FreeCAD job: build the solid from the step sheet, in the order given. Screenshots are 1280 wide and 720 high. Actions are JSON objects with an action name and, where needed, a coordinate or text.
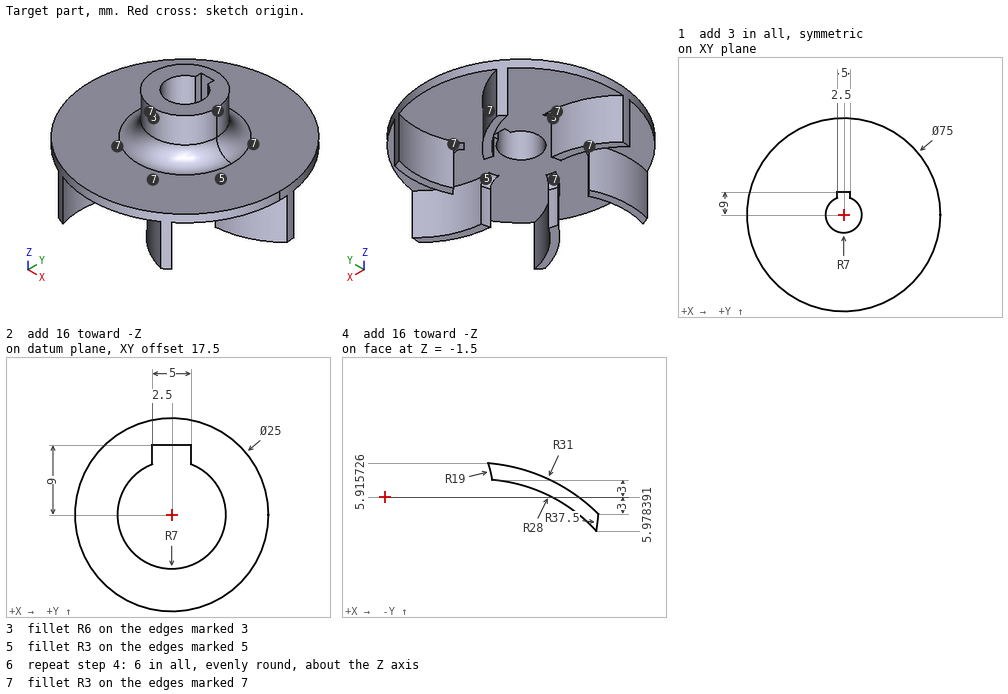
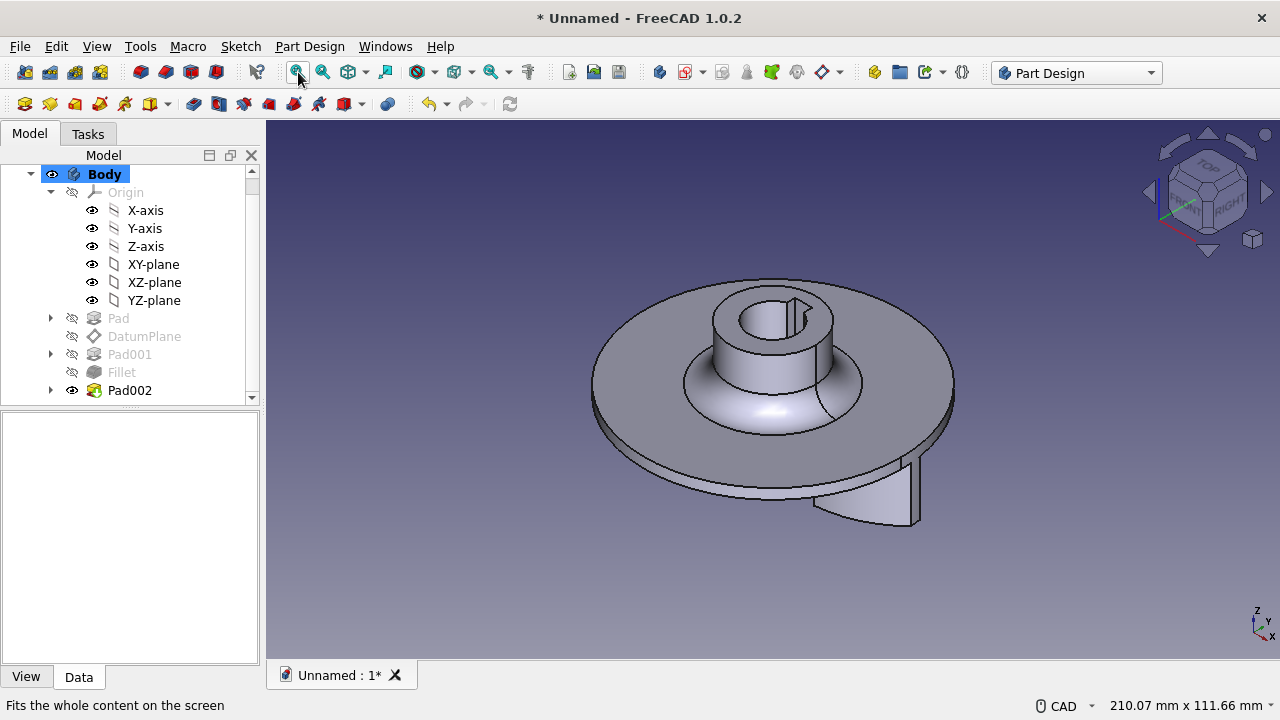
{"action": "key", "text": "2"}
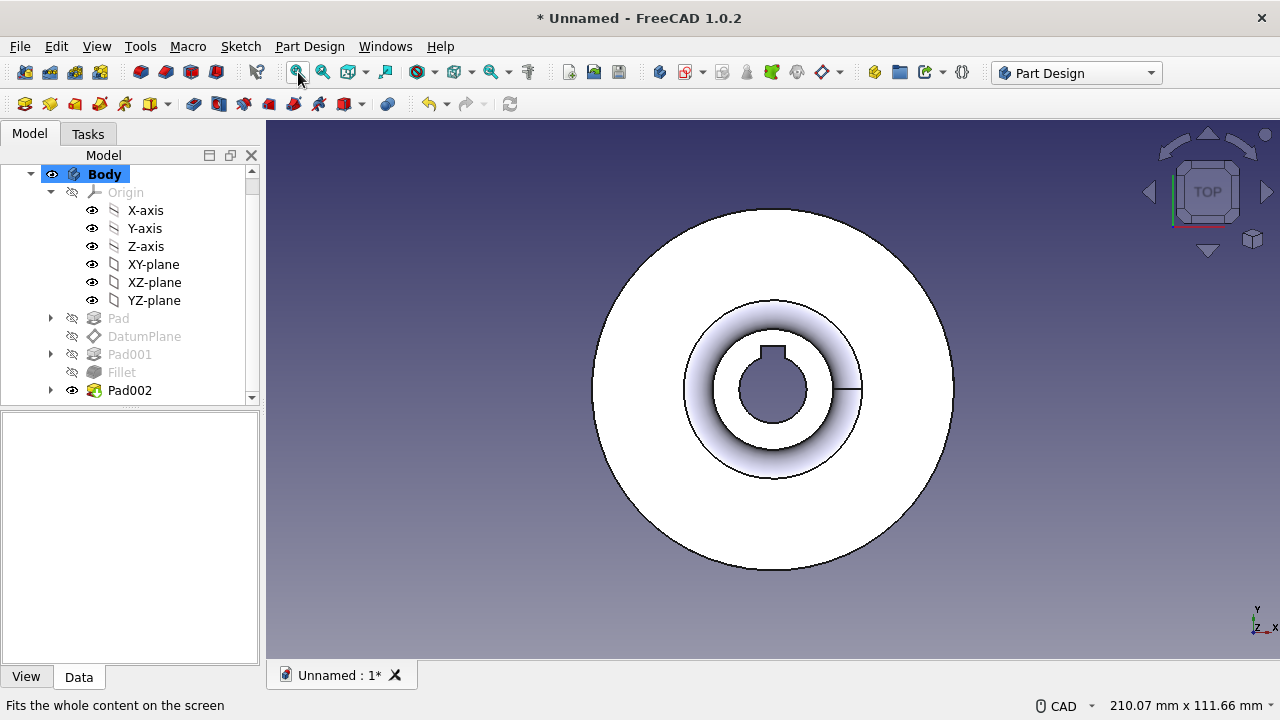
{"action": "scroll", "coordinate": [862, 410], "scroll_direction": "up", "scroll_amount": 6}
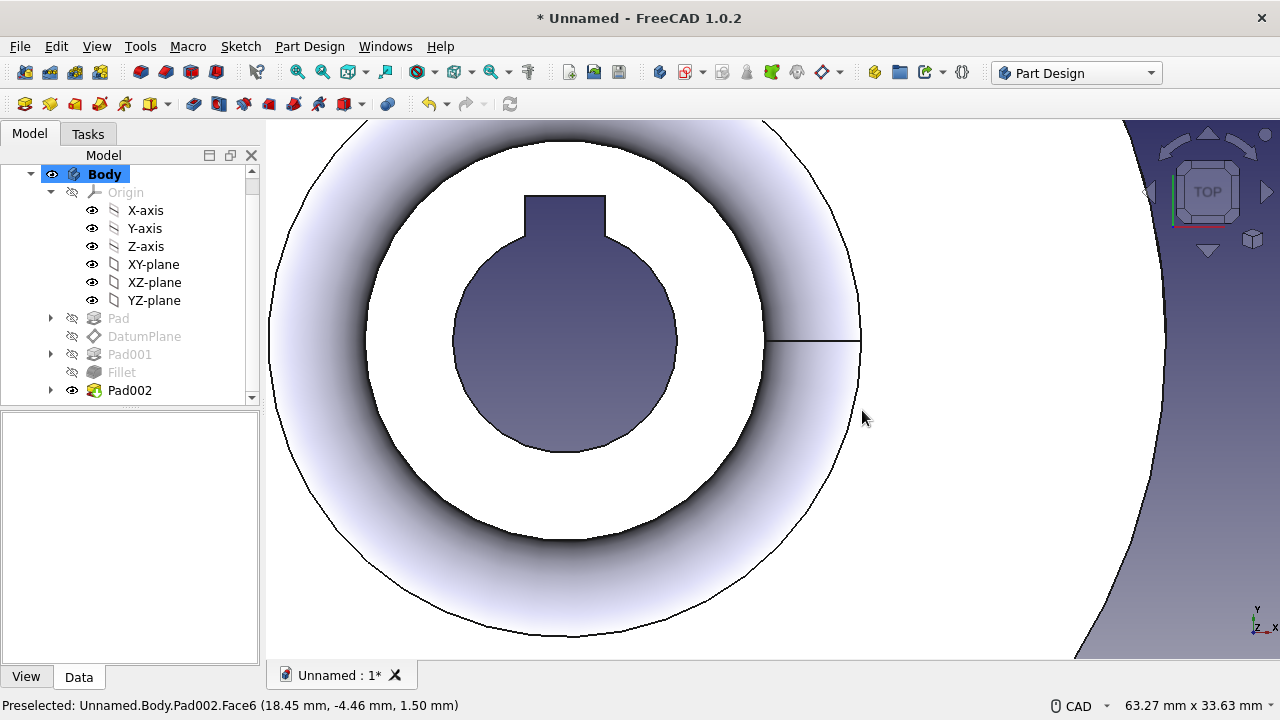
{"action": "left_click", "coordinate": [298, 72]}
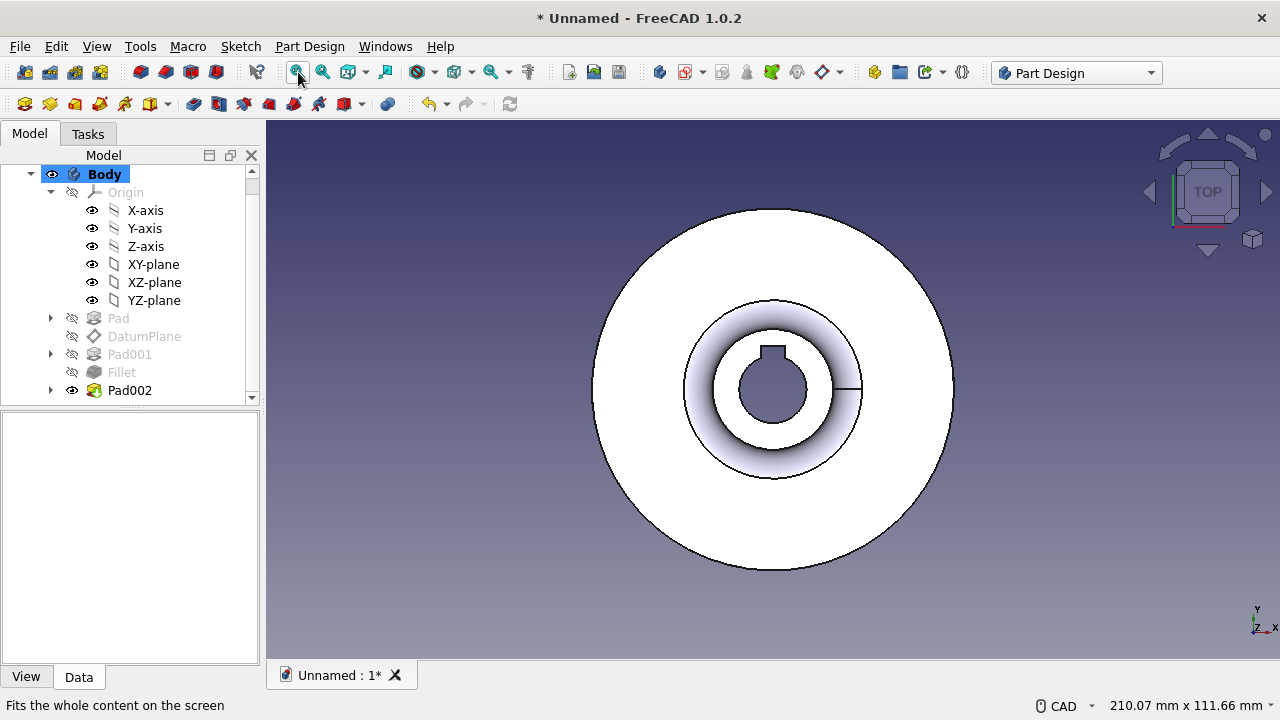
{"action": "key", "text": "1"}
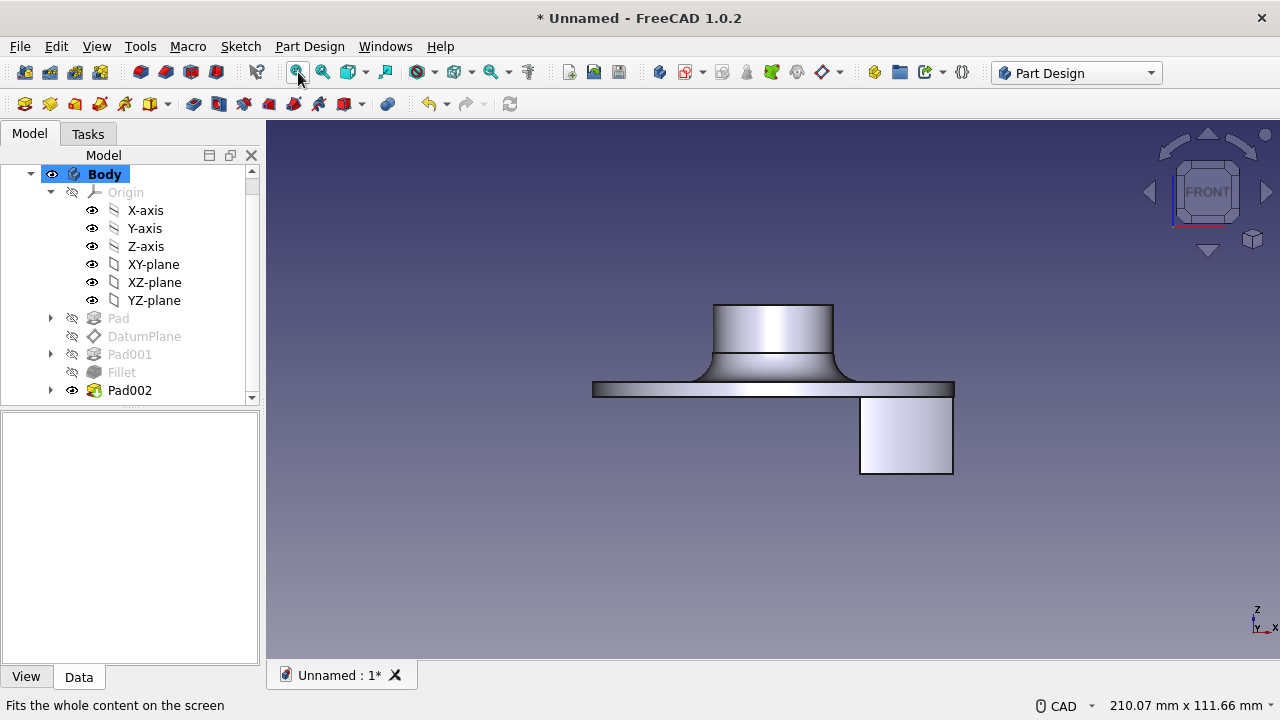
{"action": "left_click", "coordinate": [298, 72]}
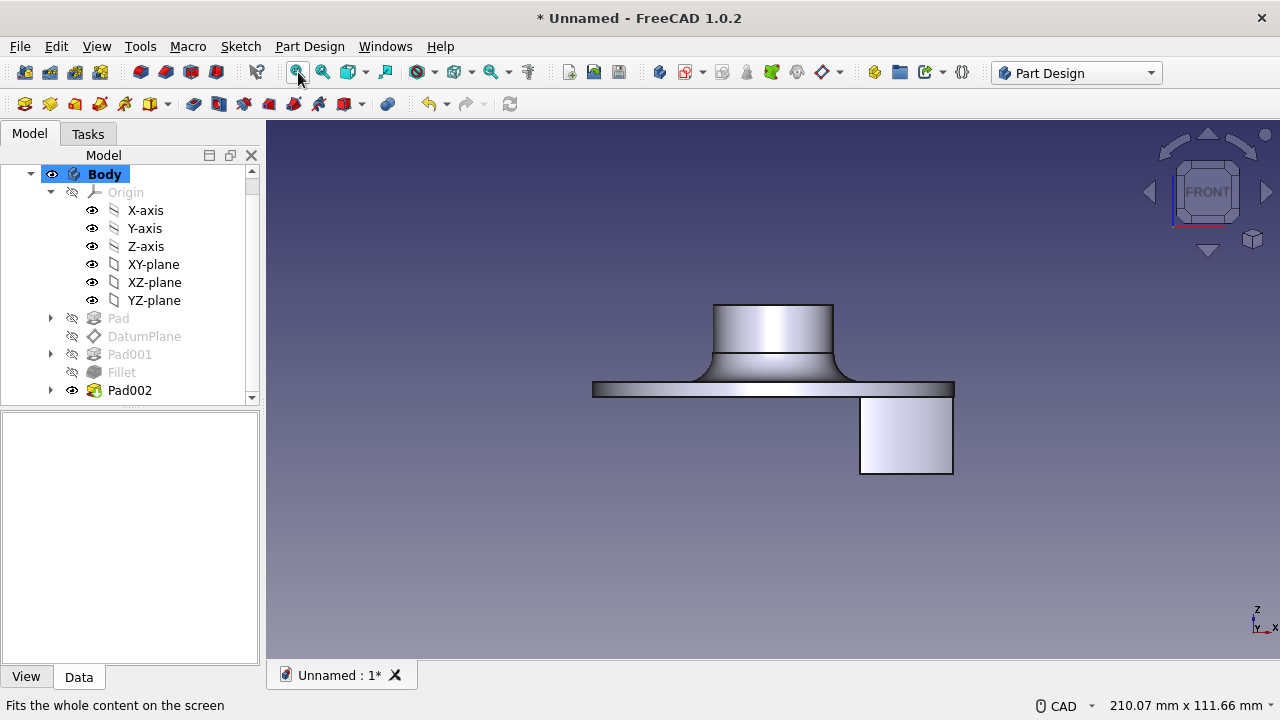
{"action": "scroll", "coordinate": [862, 396], "scroll_direction": "up", "scroll_amount": 6}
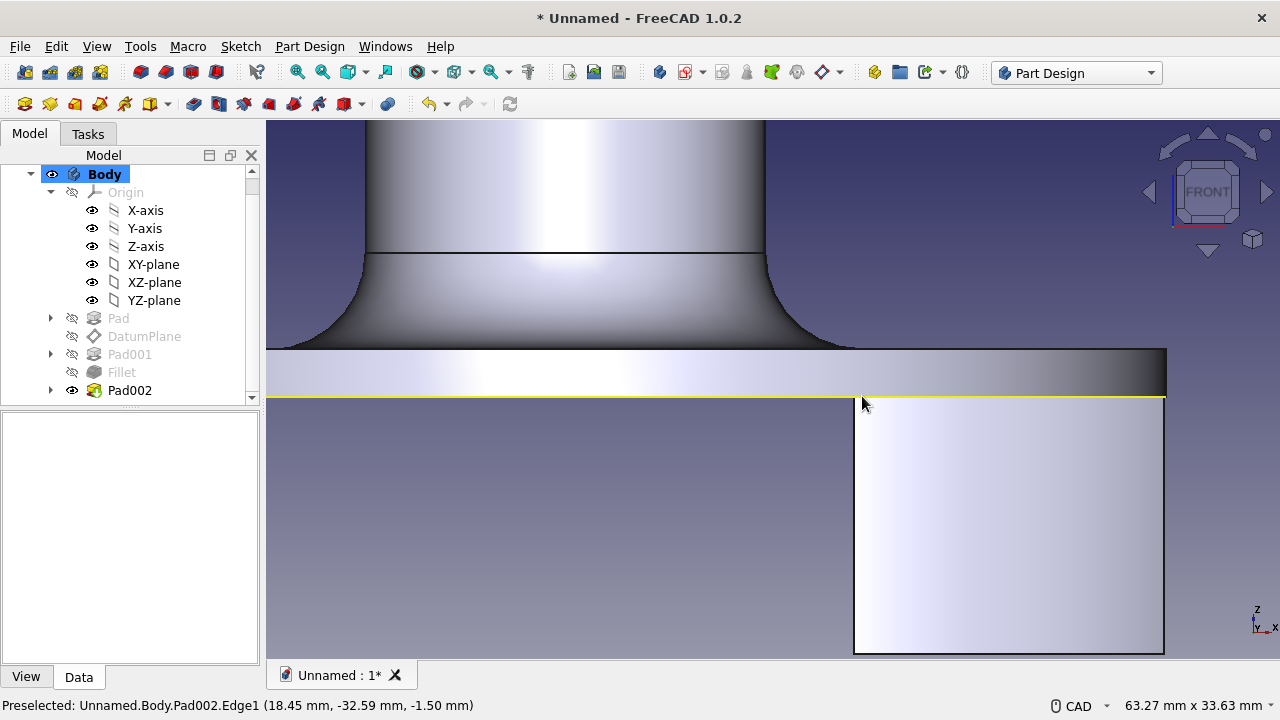
{"action": "key", "text": "v f"}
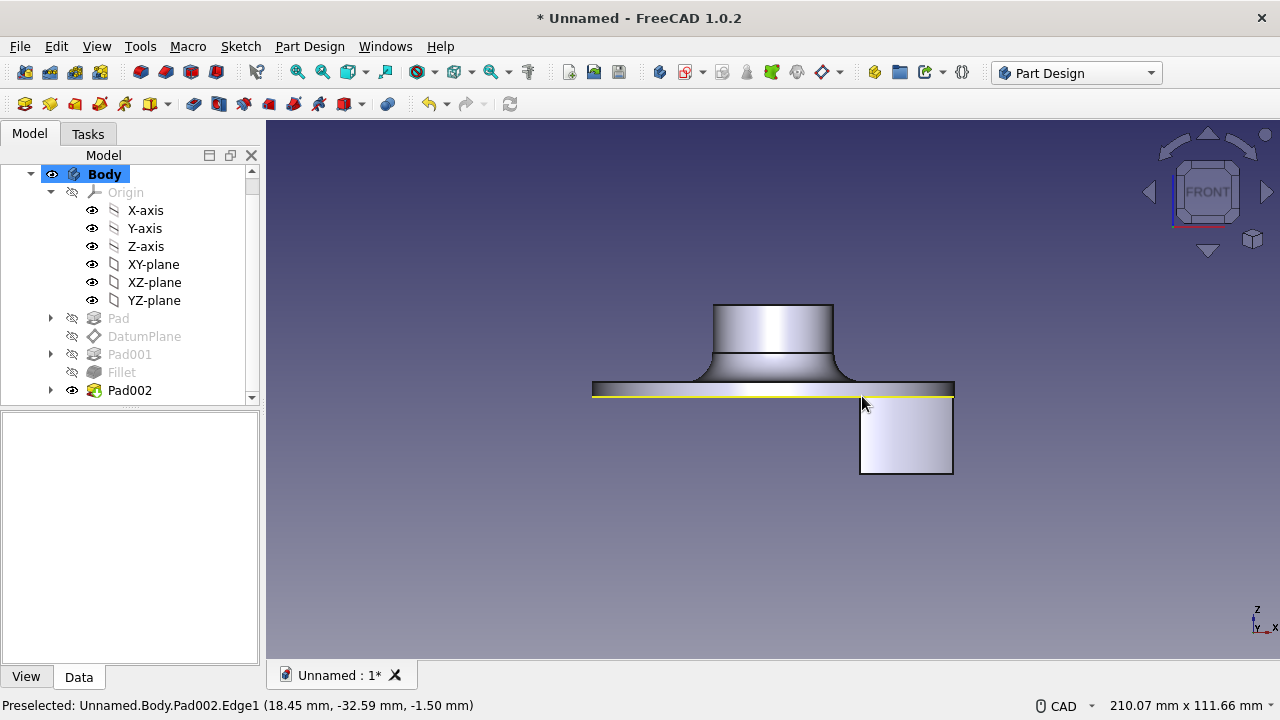
{"action": "key", "text": "3"}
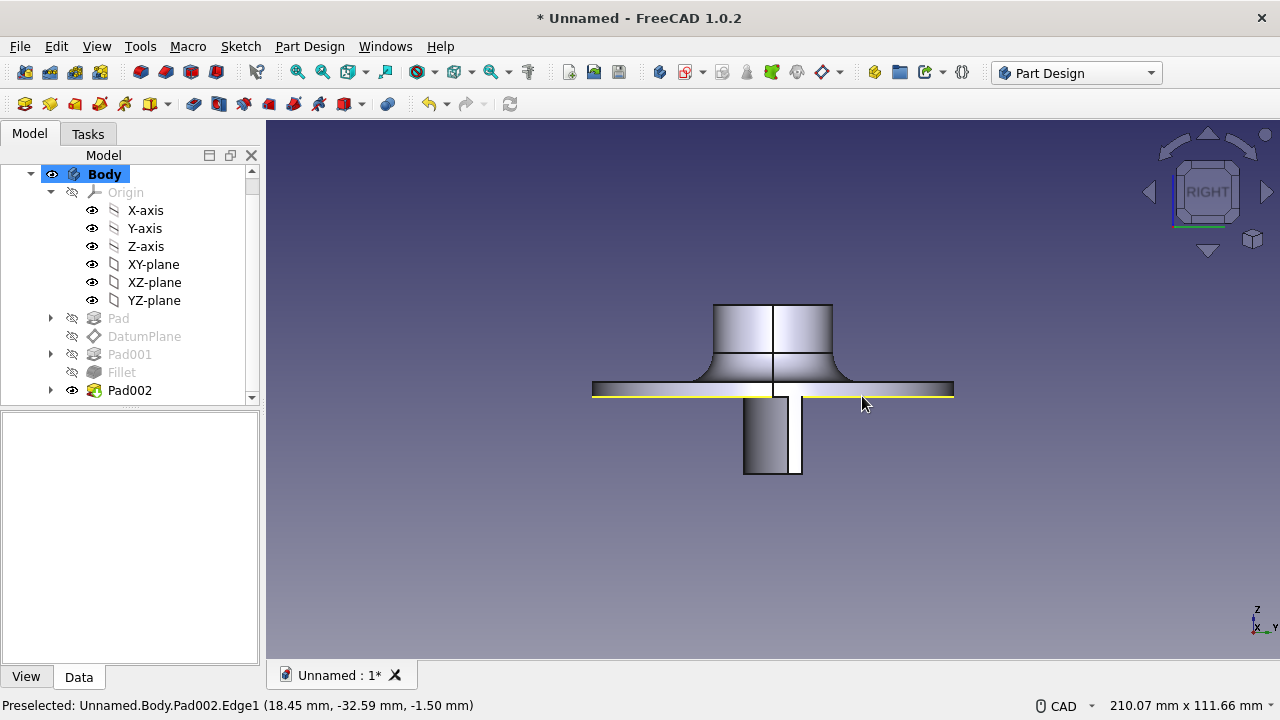
{"action": "left_click", "coordinate": [298, 72]}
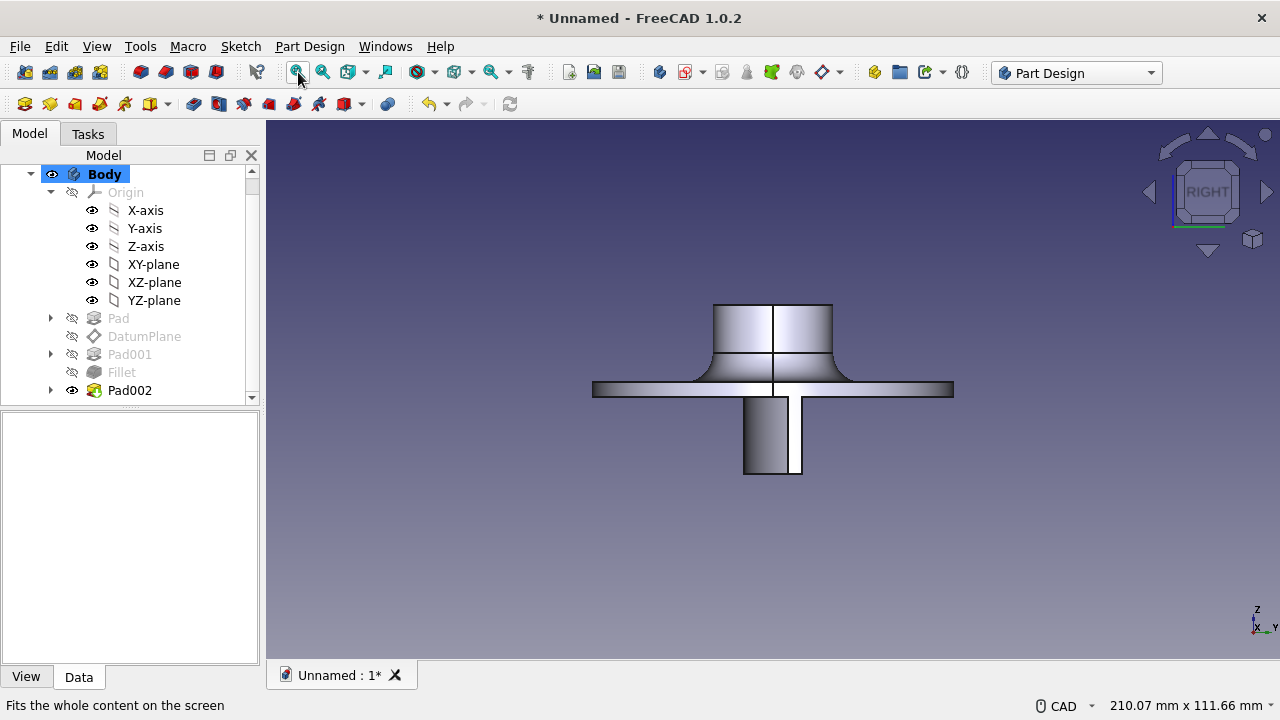
{"action": "scroll", "coordinate": [751, 396], "scroll_direction": "up", "scroll_amount": 6}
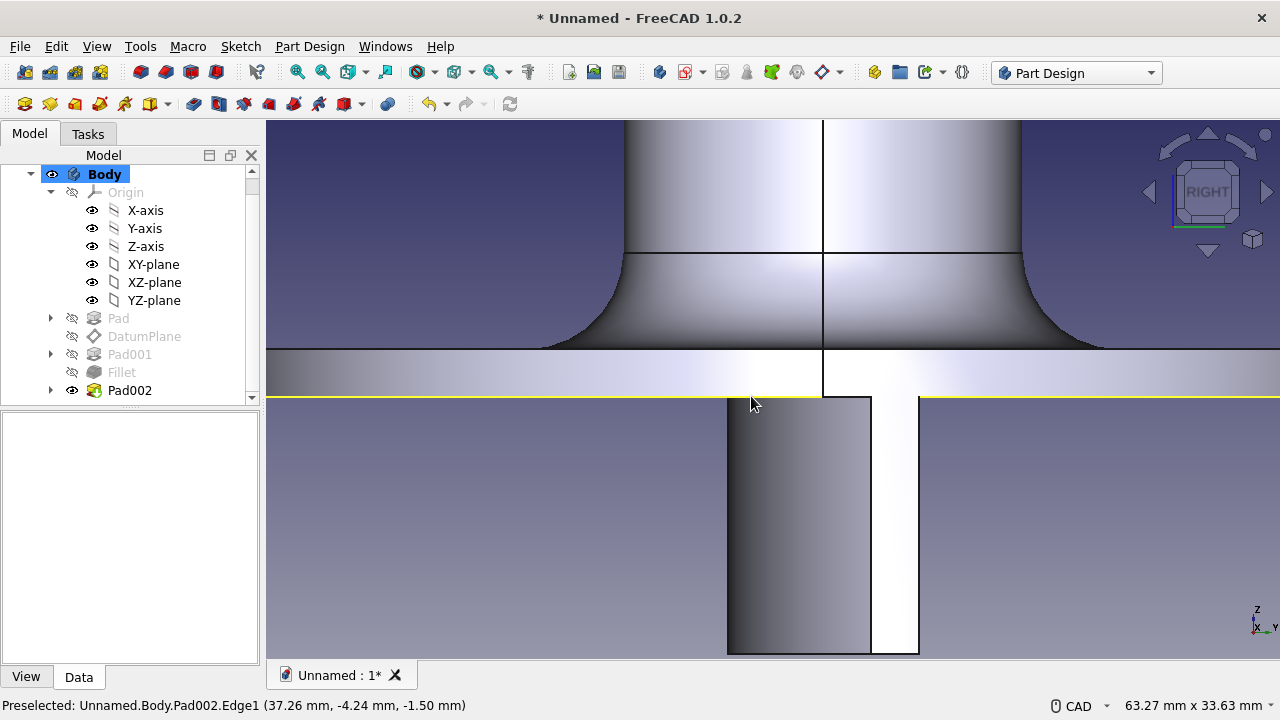
{"action": "key", "text": "v f"}